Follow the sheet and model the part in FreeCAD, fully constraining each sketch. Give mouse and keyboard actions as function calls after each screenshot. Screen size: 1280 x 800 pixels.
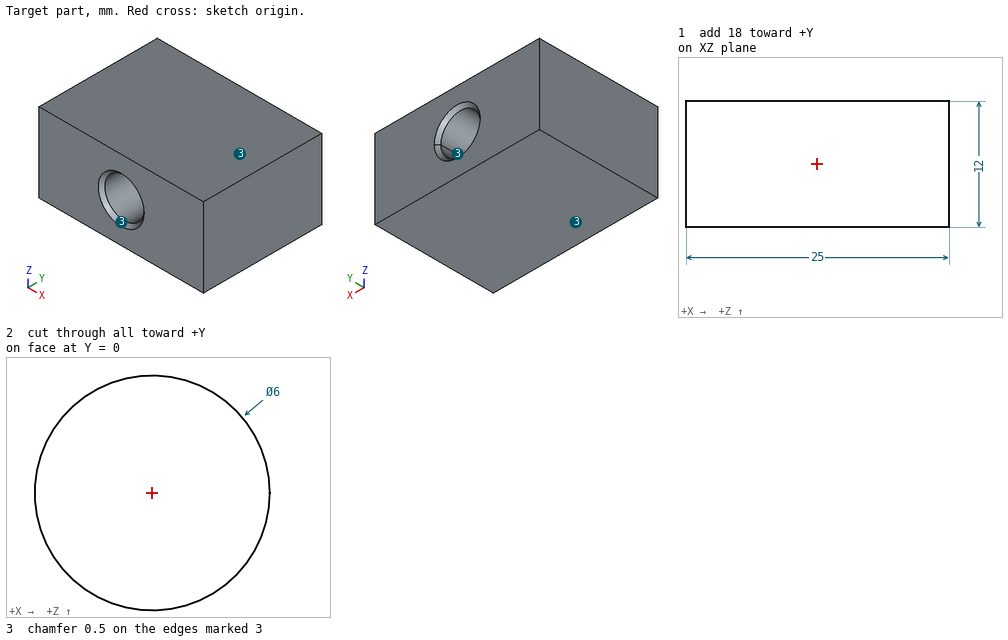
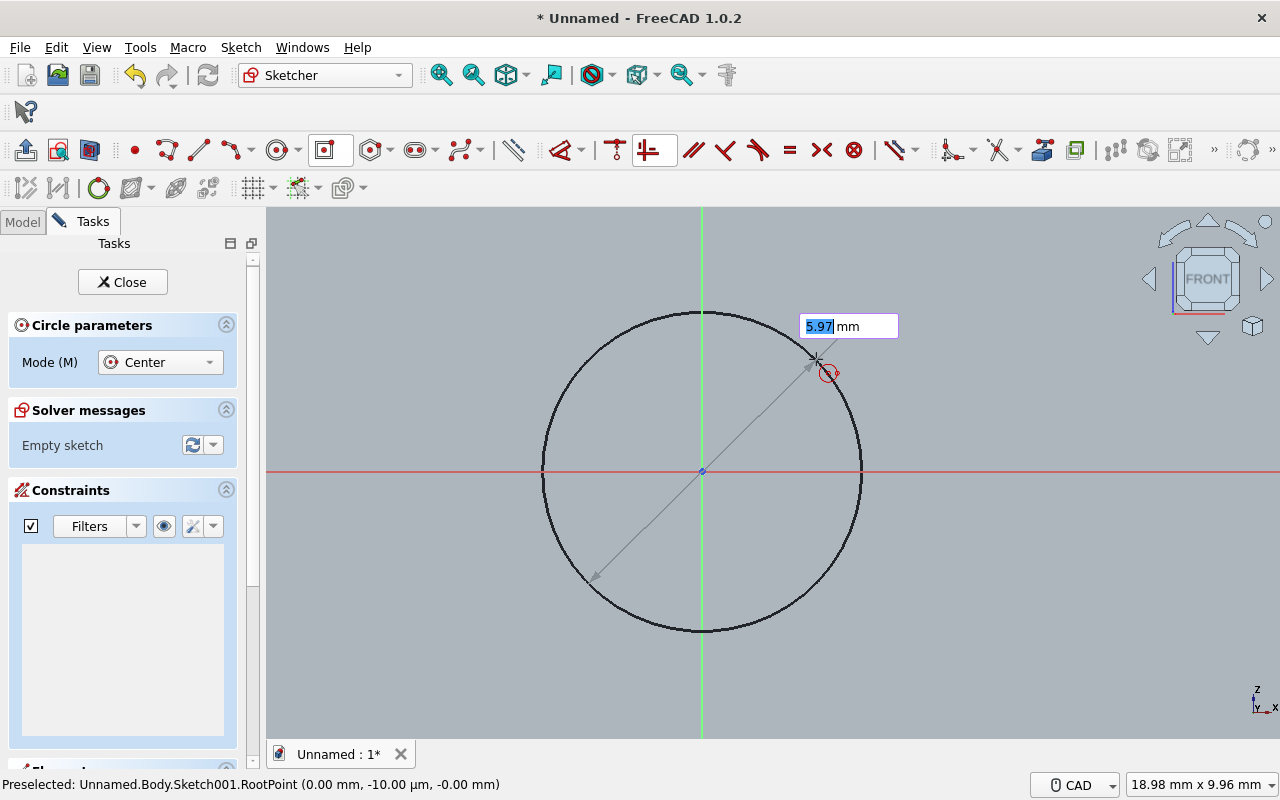
text(6)
key(Return)
key(Escape)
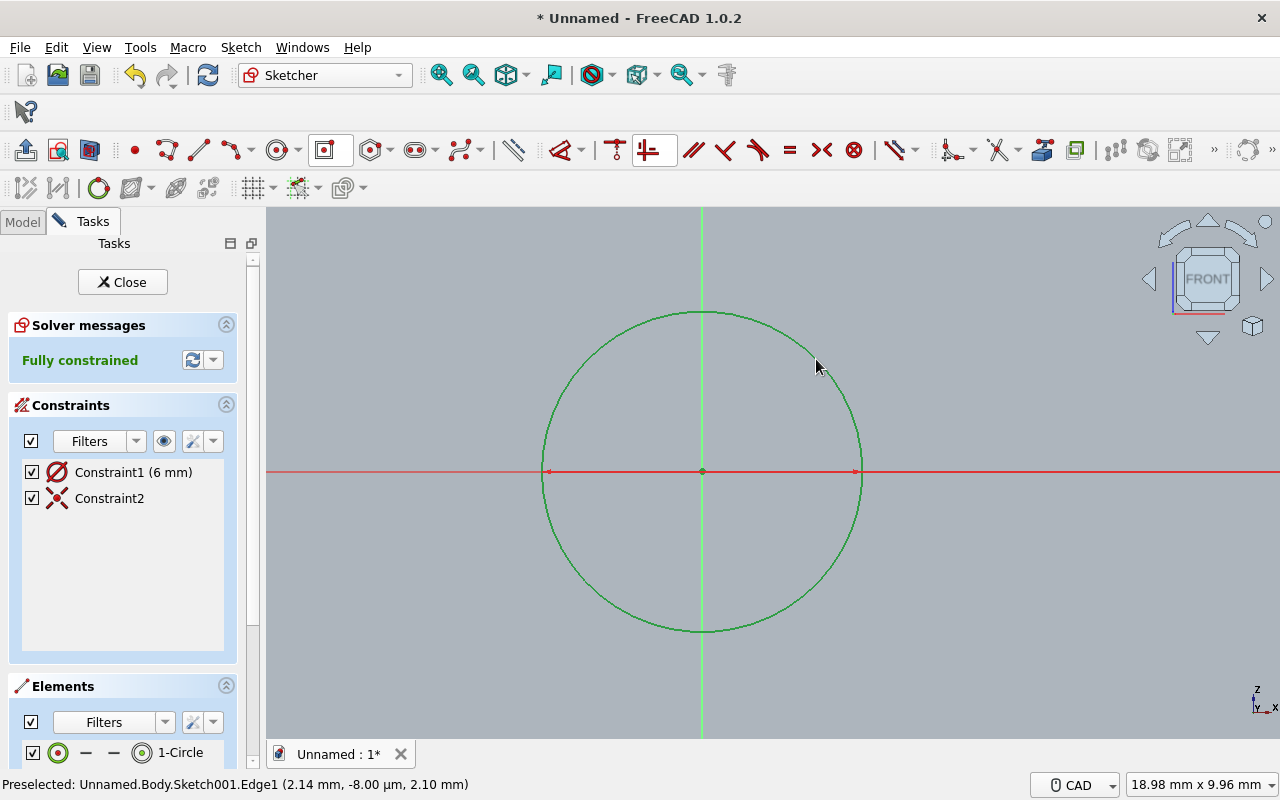
click(123, 282)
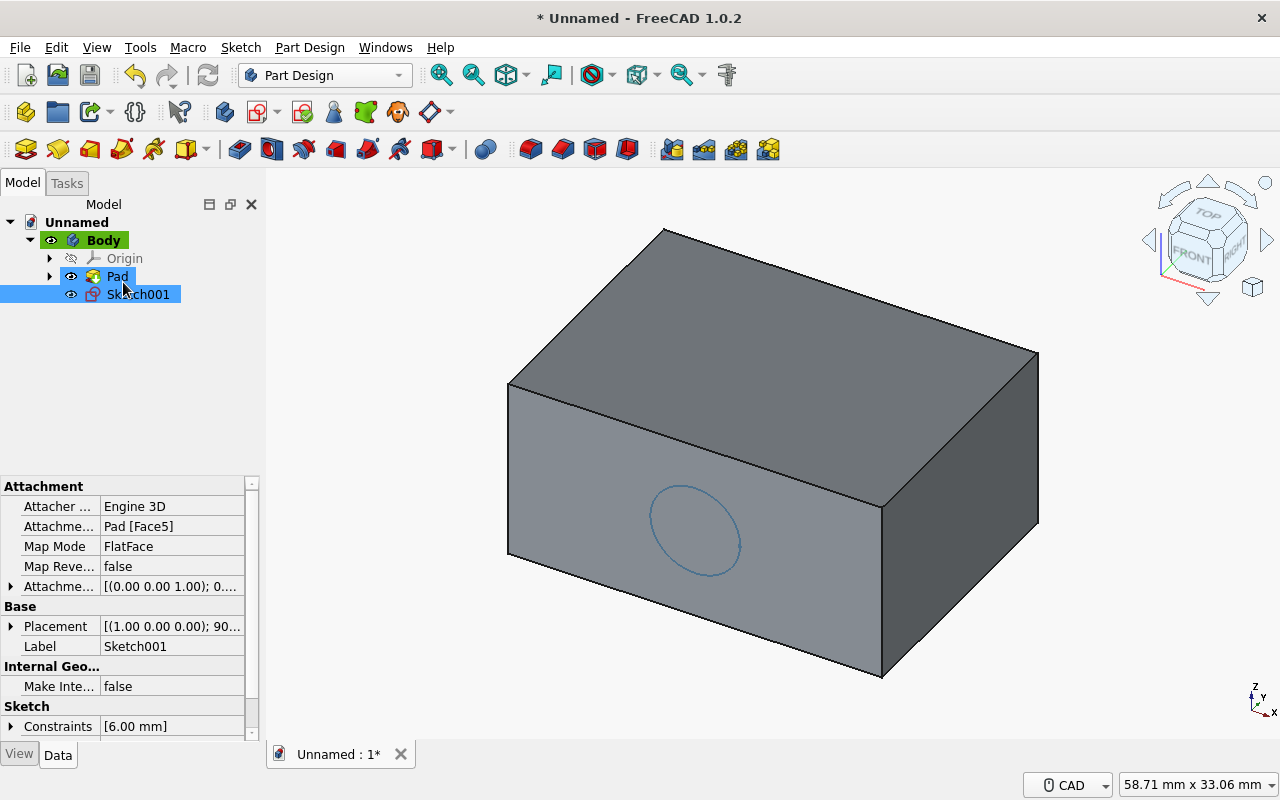
click(240, 150)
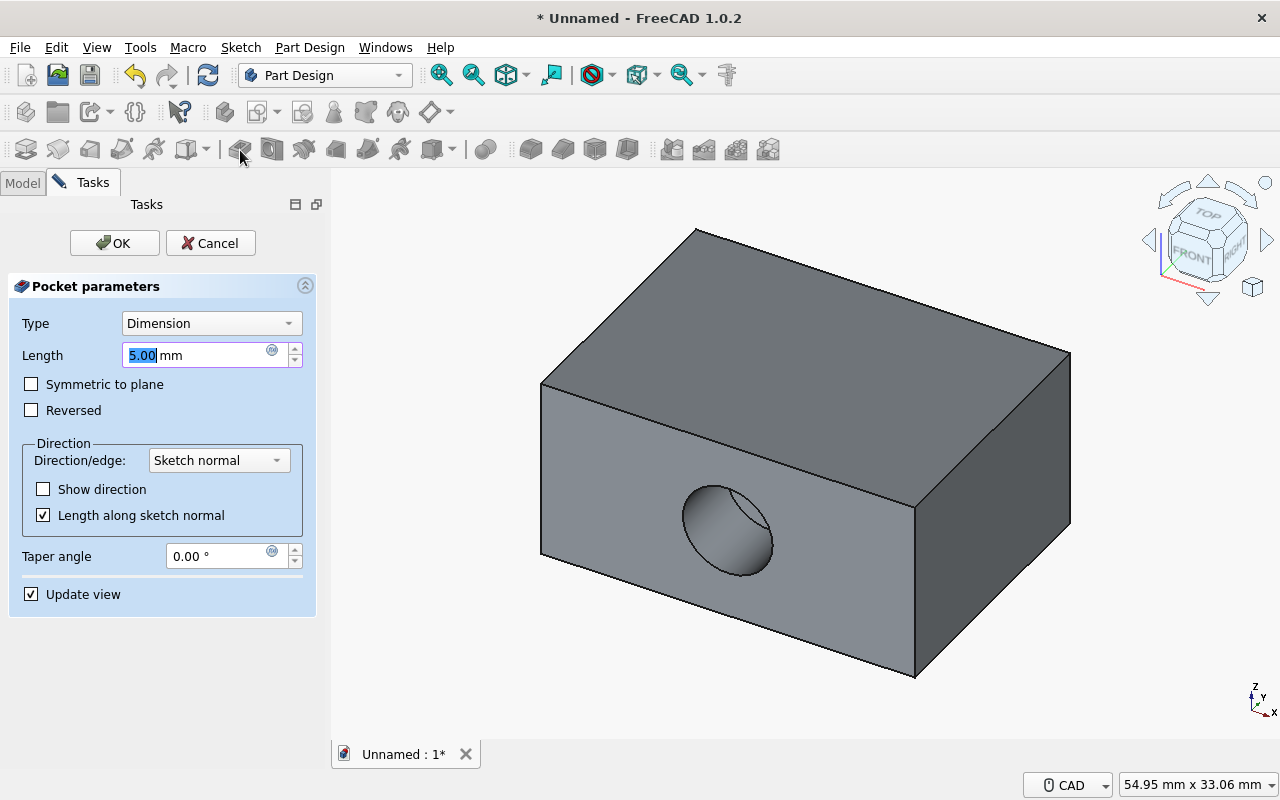
click(212, 324)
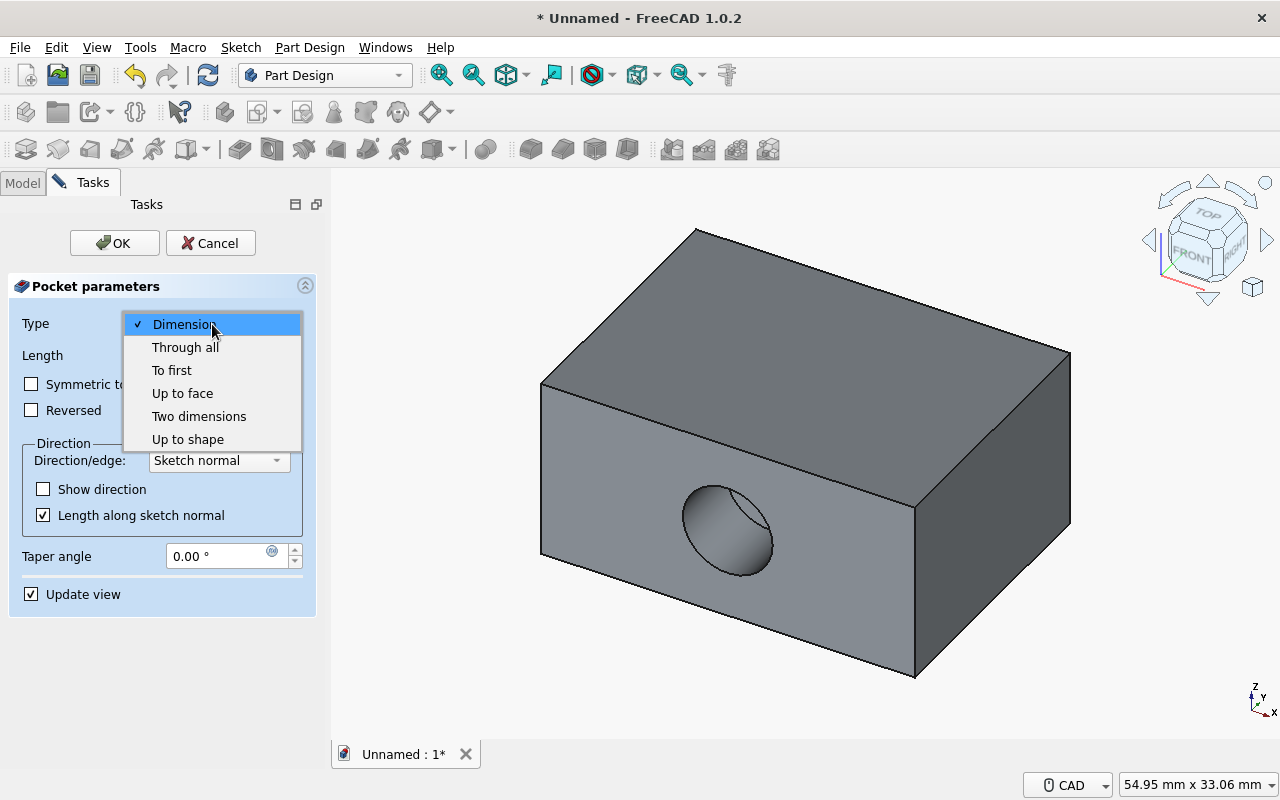
click(212, 348)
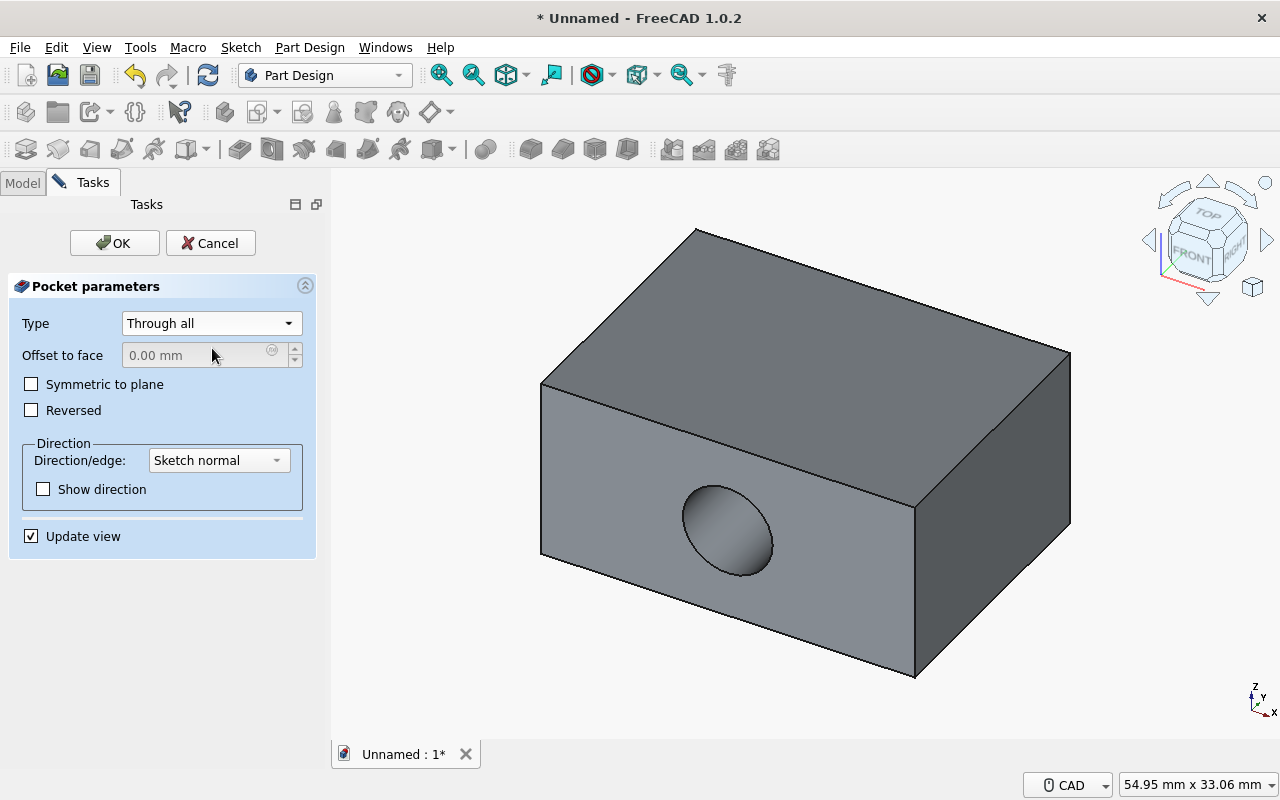
click(115, 243)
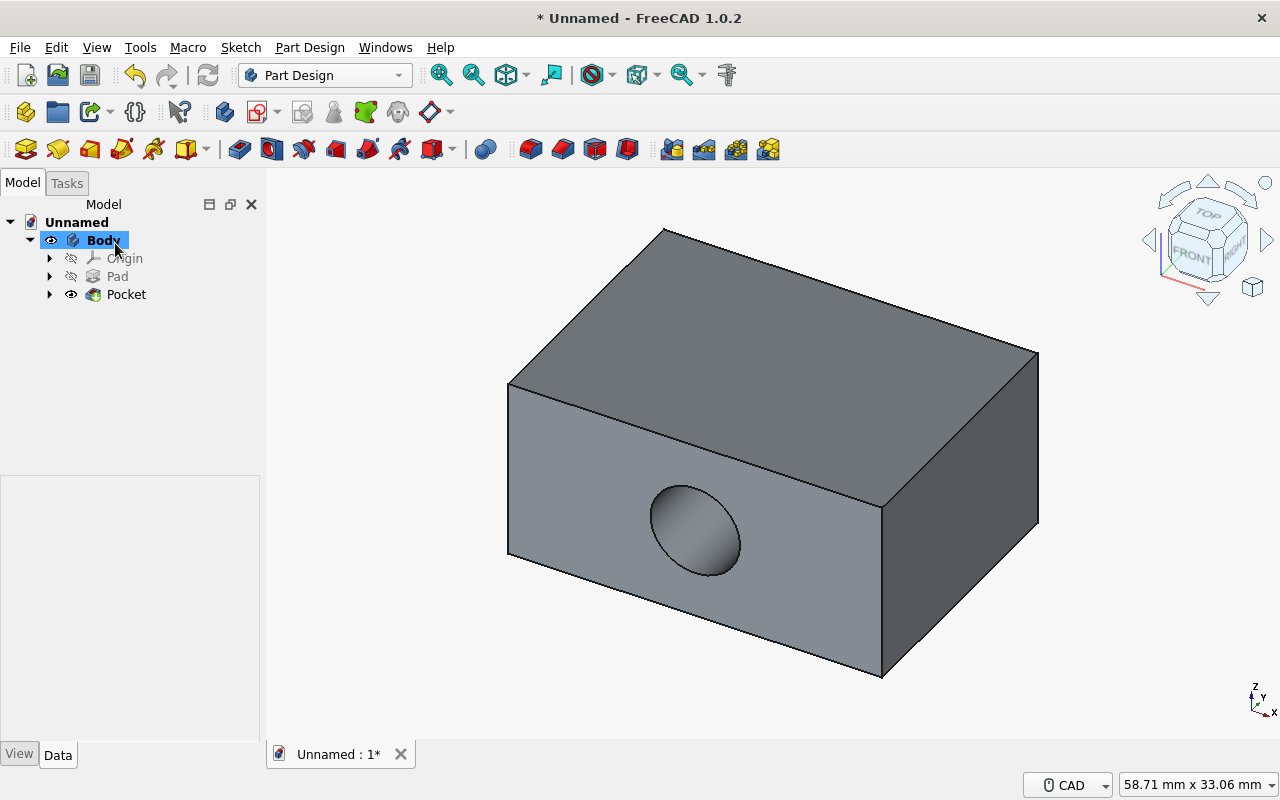
click(650, 515)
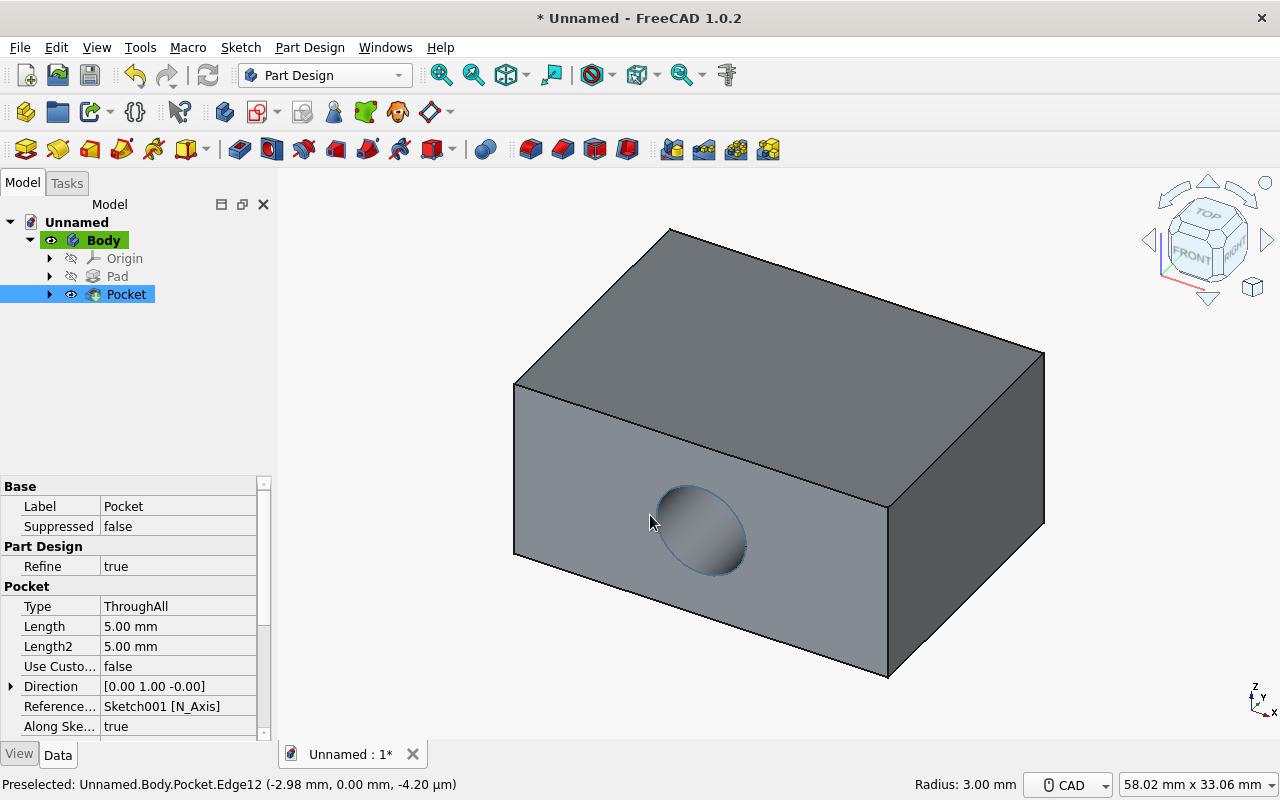
key(0)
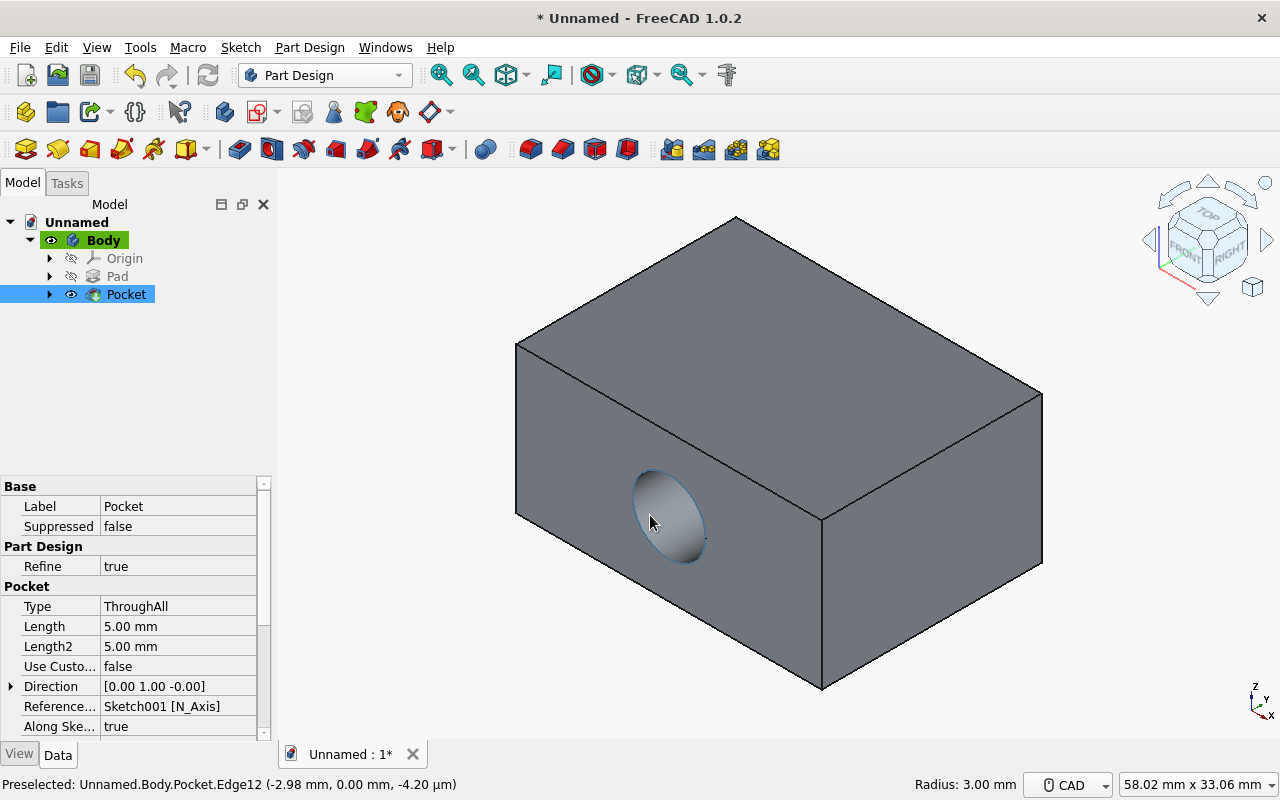
key(2)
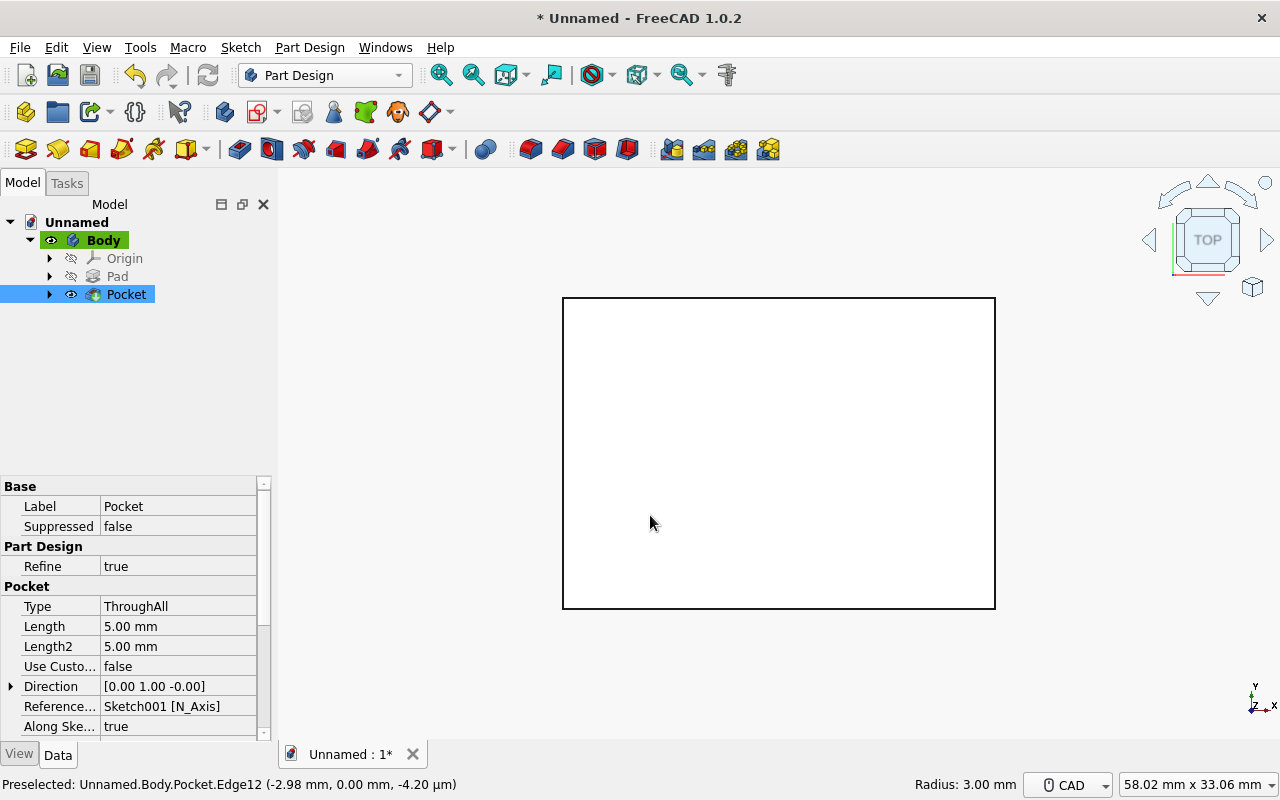
key(1)